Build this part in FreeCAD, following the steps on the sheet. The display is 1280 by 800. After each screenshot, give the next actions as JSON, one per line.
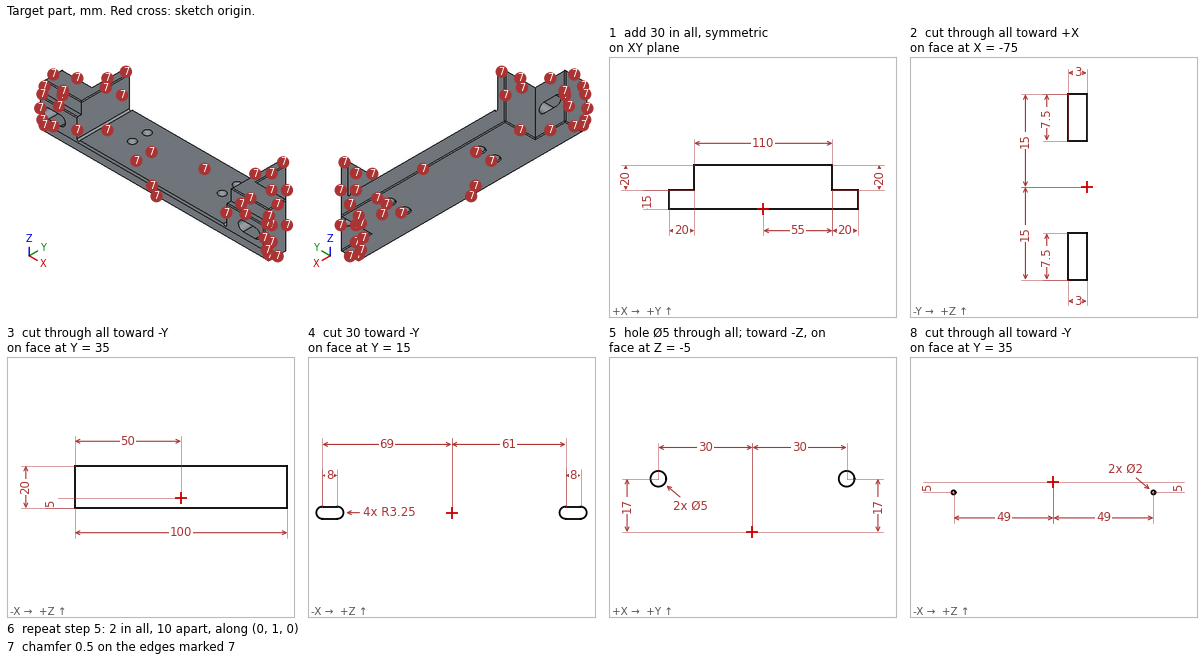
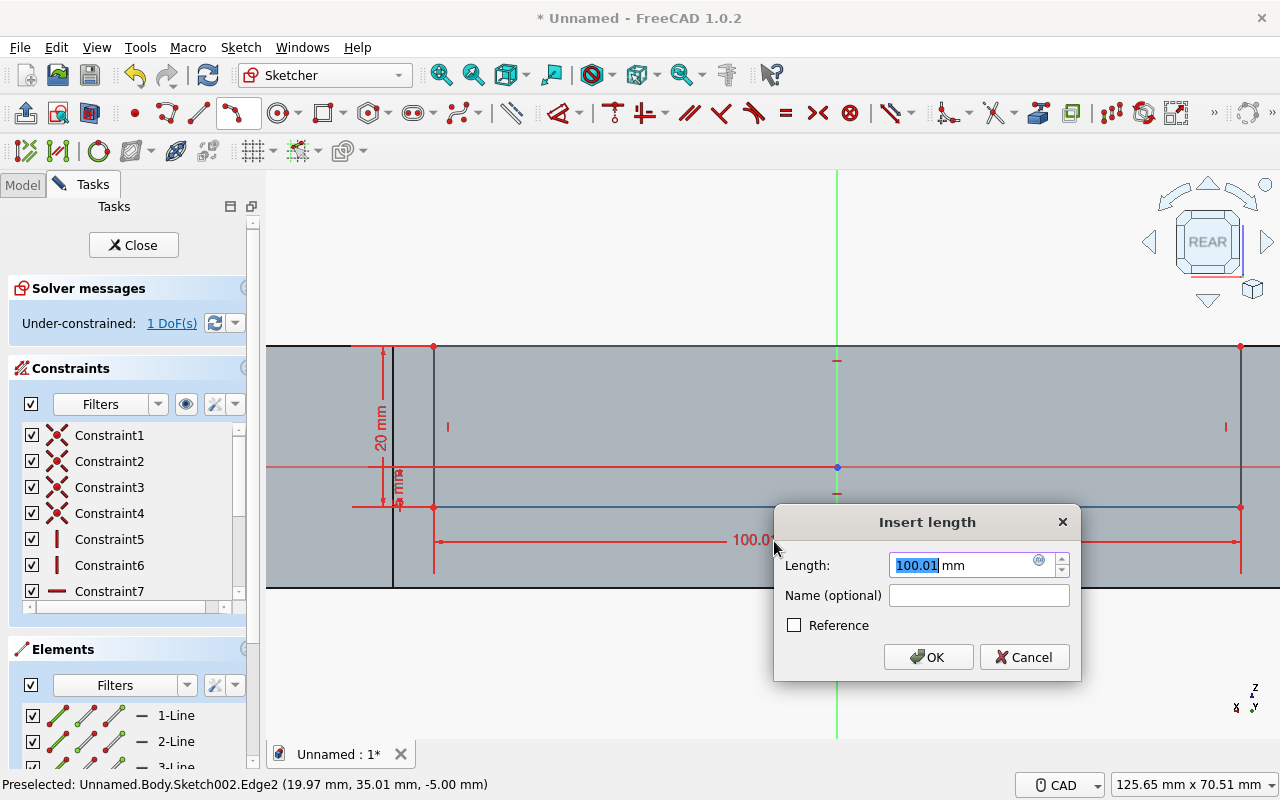
{"action": "type", "text": "100"}
{"action": "key", "text": "Return"}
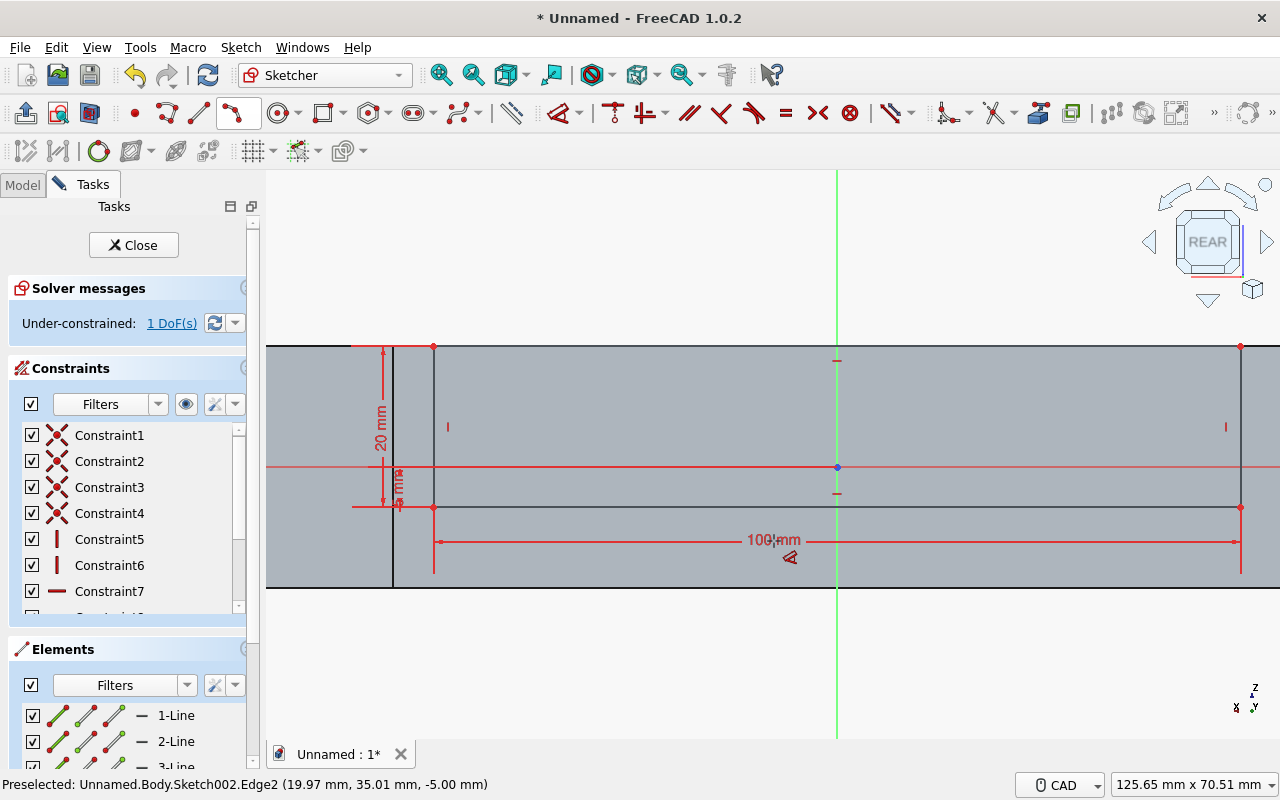
{"action": "left_click", "coordinate": [434, 346]}
{"action": "left_click", "coordinate": [636, 312]}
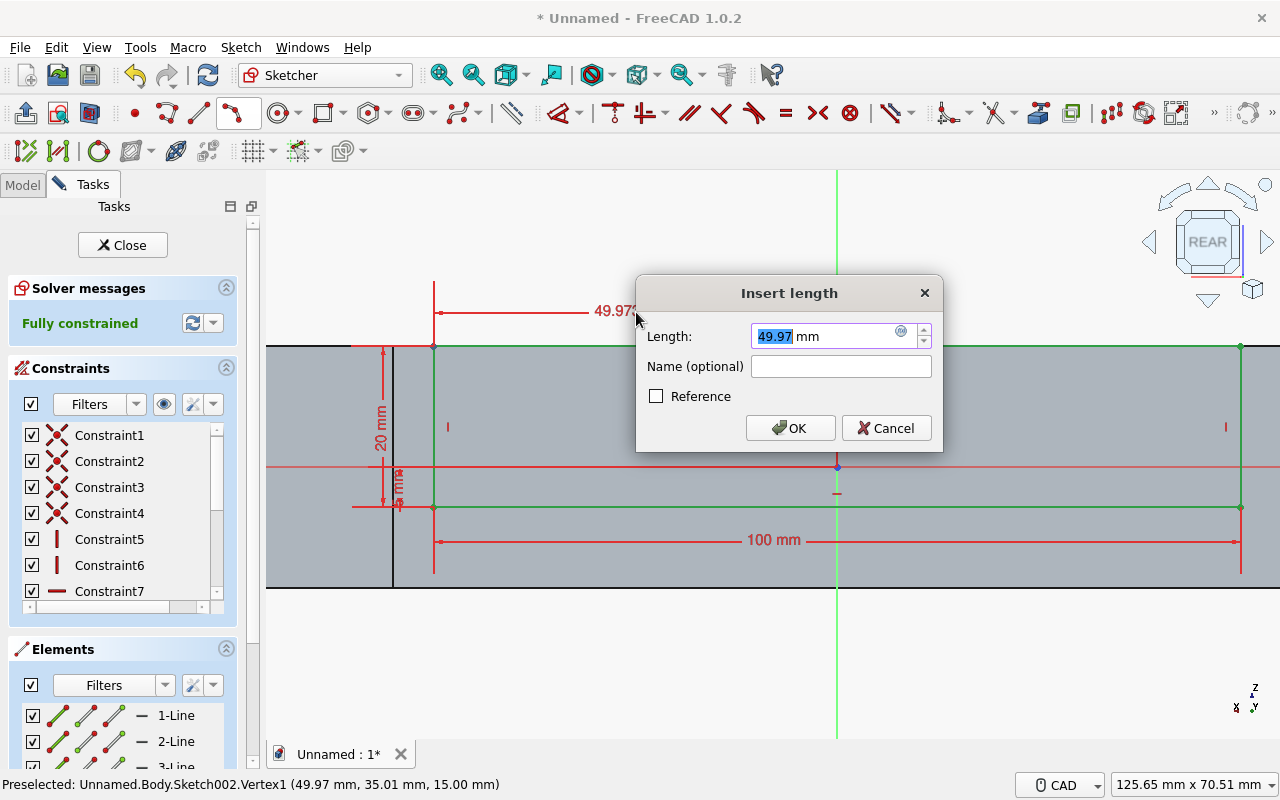
{"action": "type", "text": "50"}
{"action": "key", "text": "Return"}
{"action": "key", "text": "Escape"}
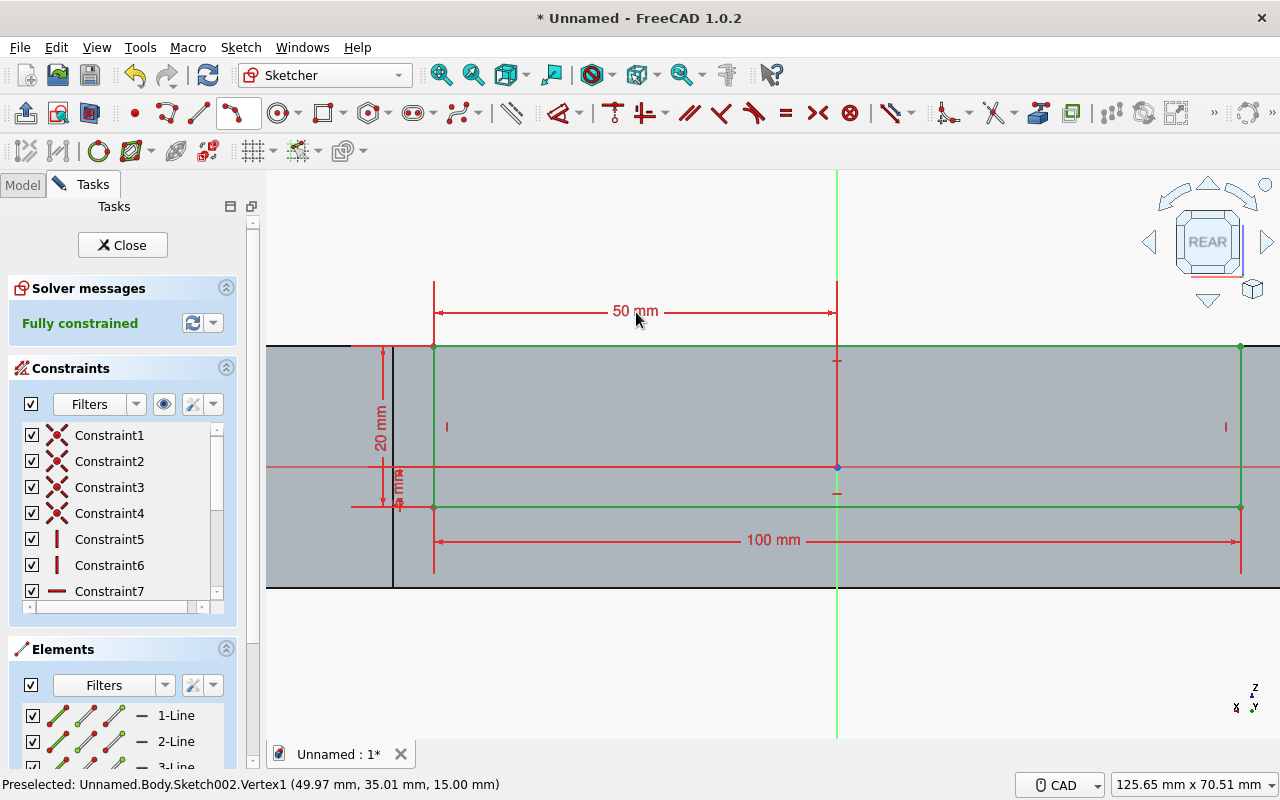
{"action": "left_click", "coordinate": [123, 245]}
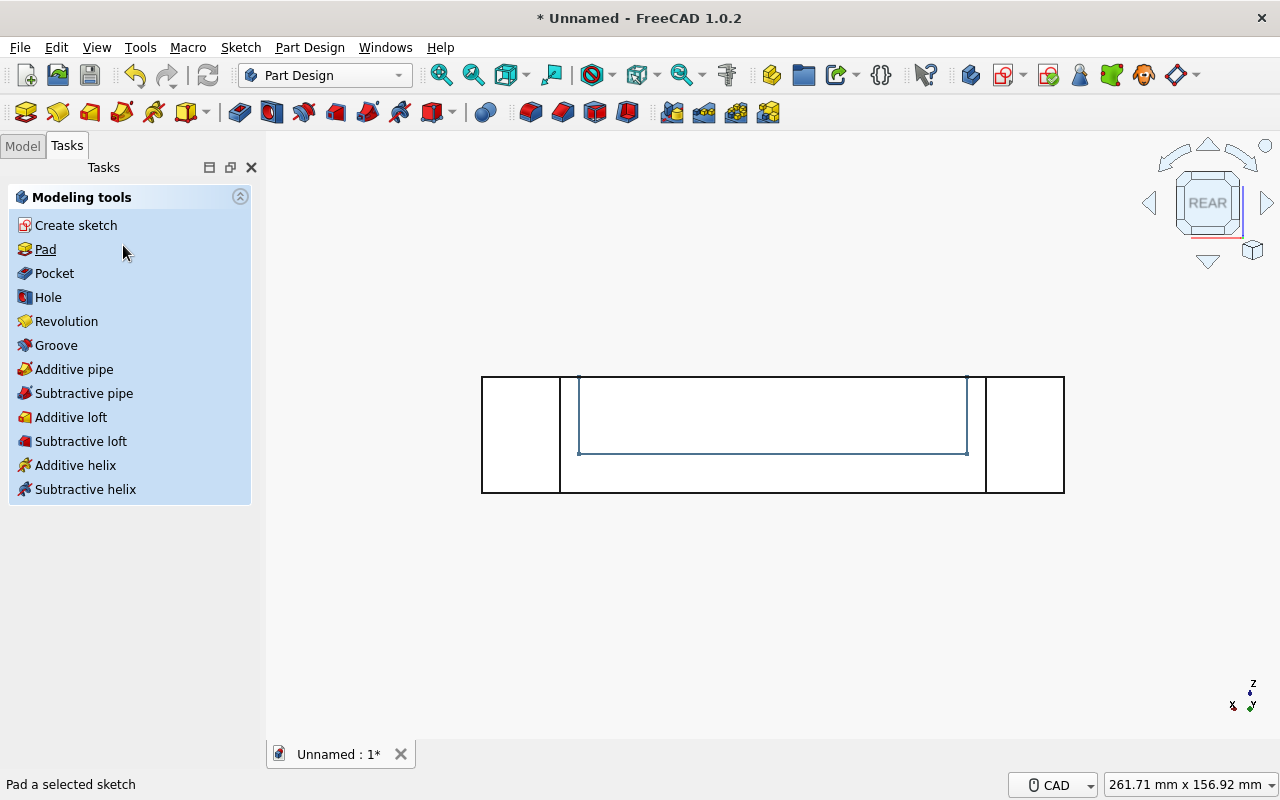
{"action": "left_click", "coordinate": [240, 112]}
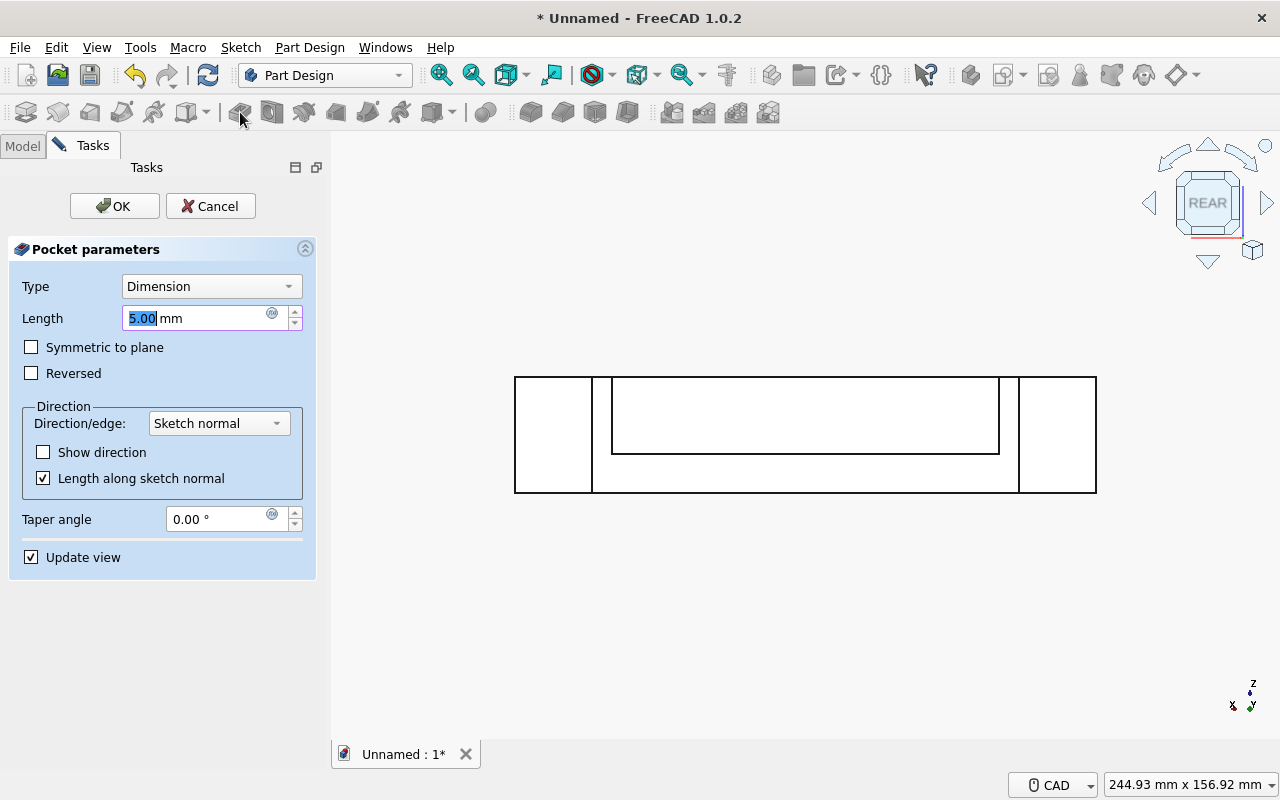
{"action": "left_click", "coordinate": [212, 286]}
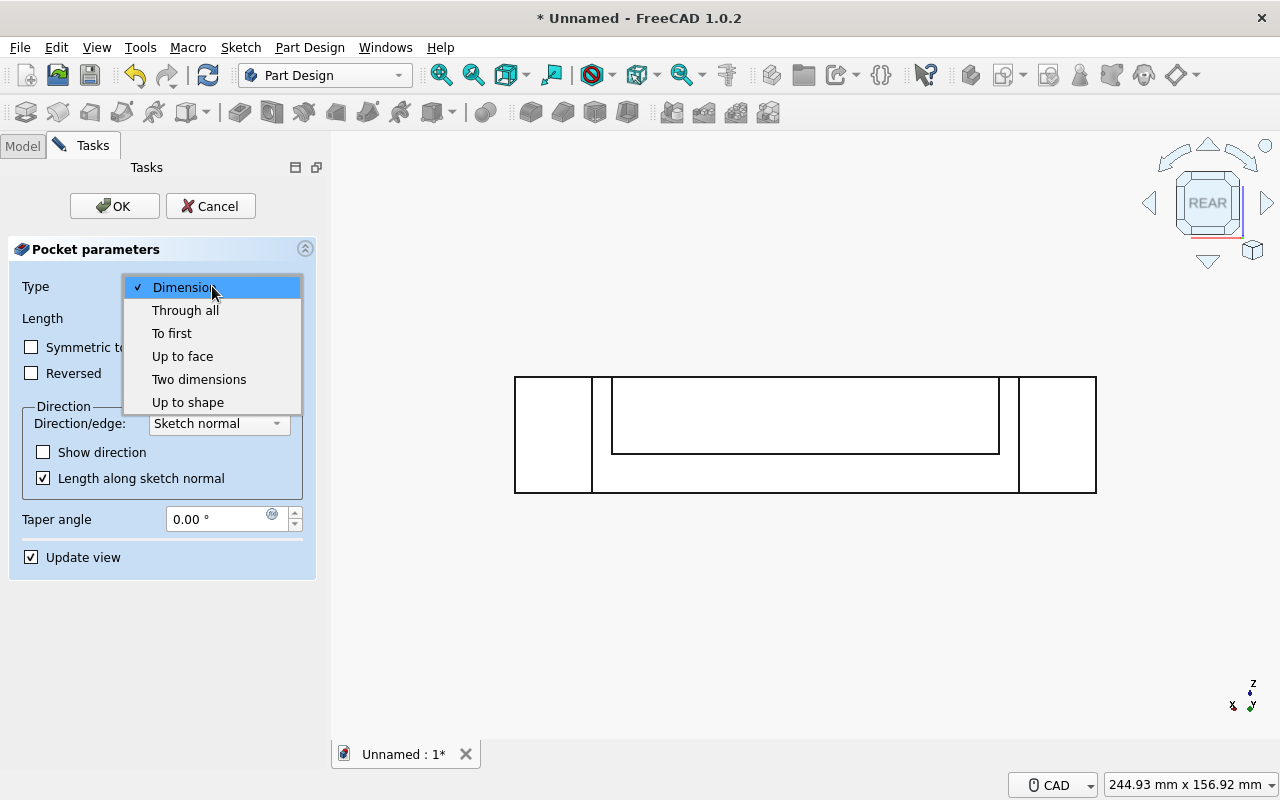
{"action": "left_click", "coordinate": [212, 310]}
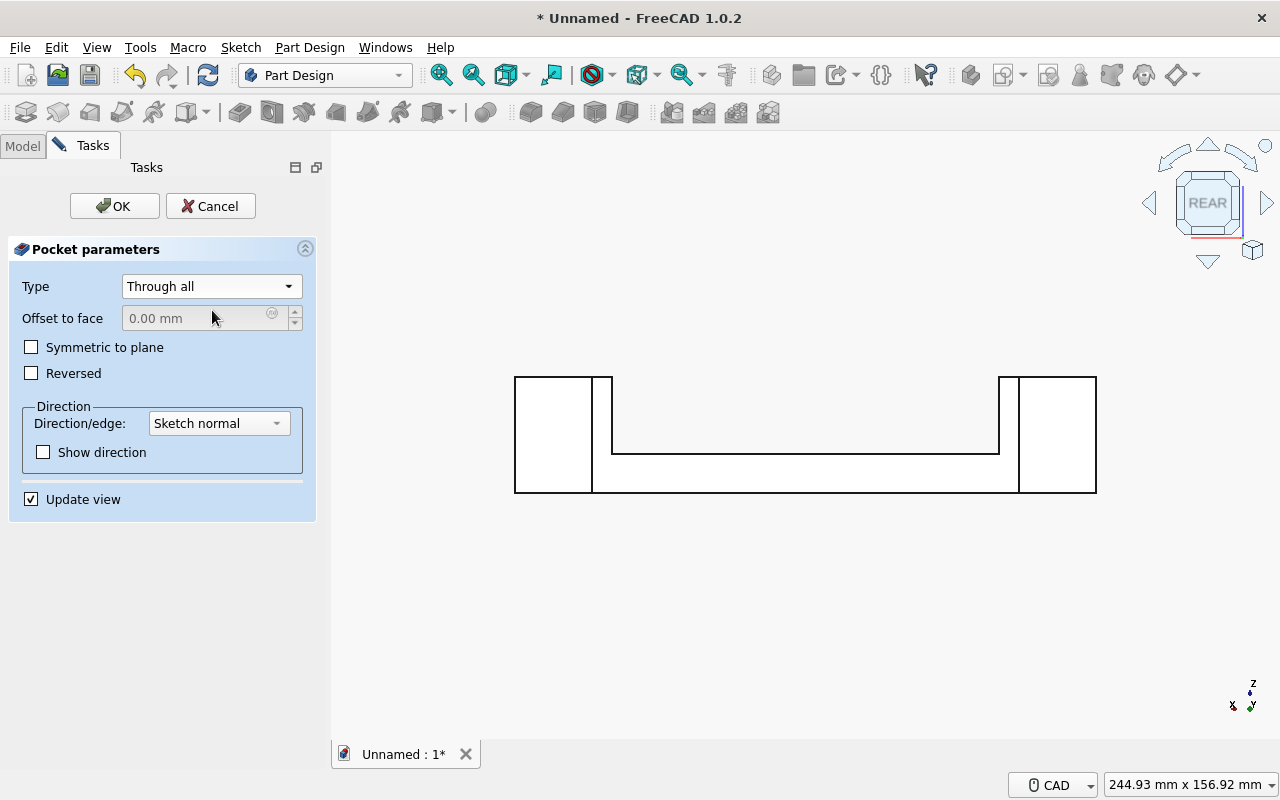
{"action": "left_click", "coordinate": [115, 206]}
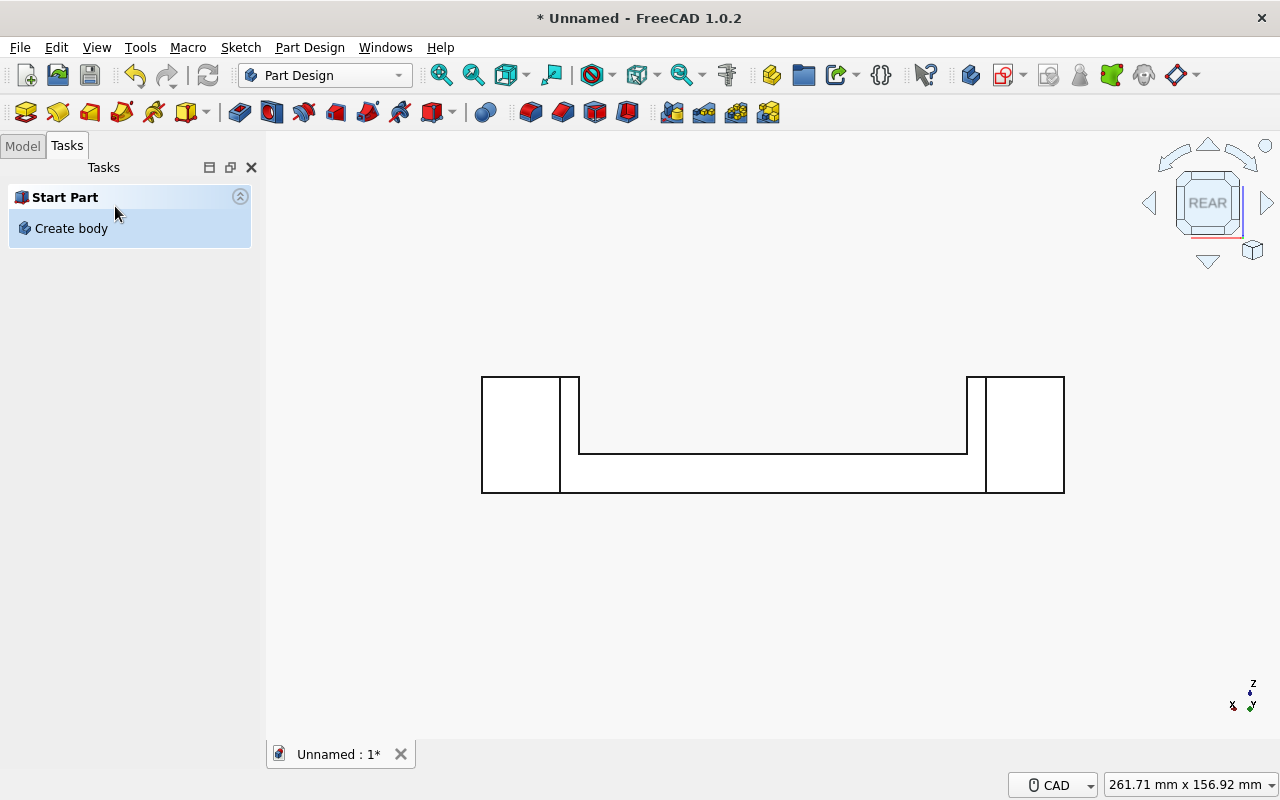
{"action": "left_click", "coordinate": [521, 417]}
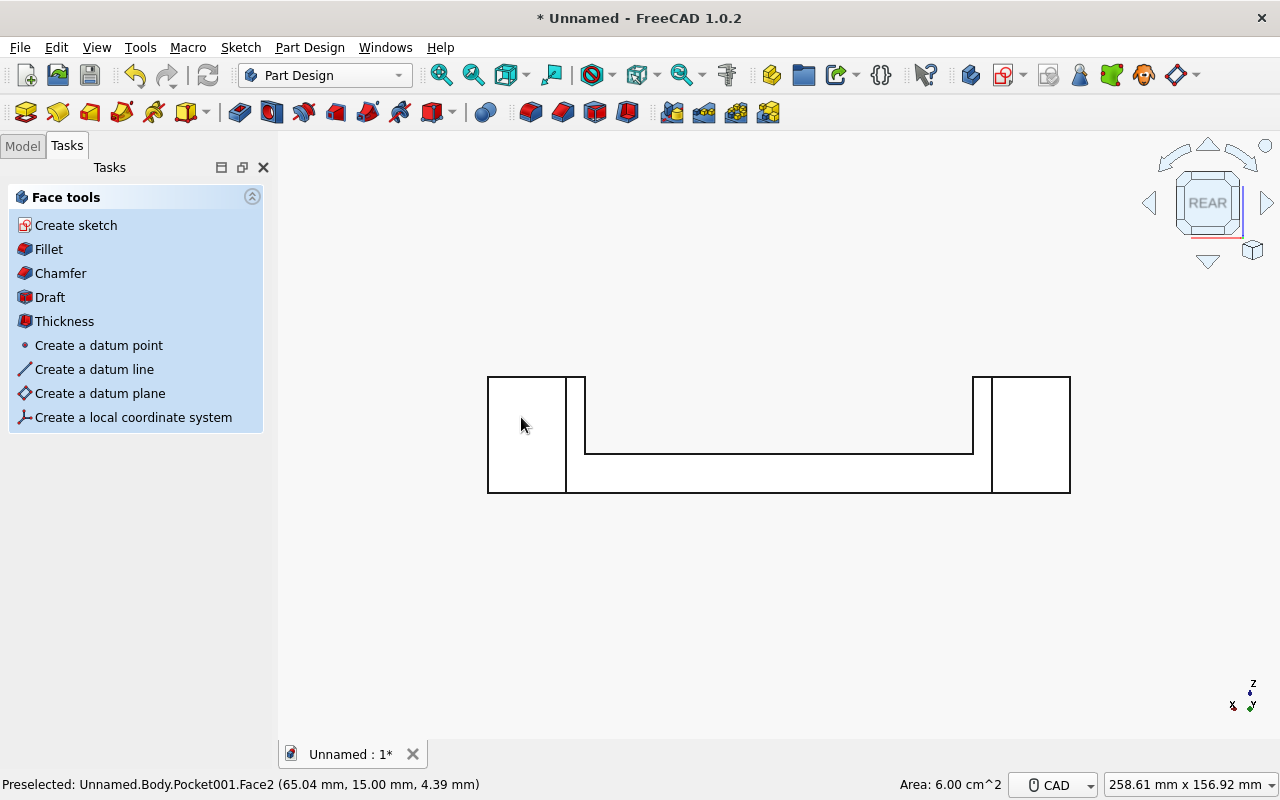
{"action": "left_click", "coordinate": [1004, 76]}